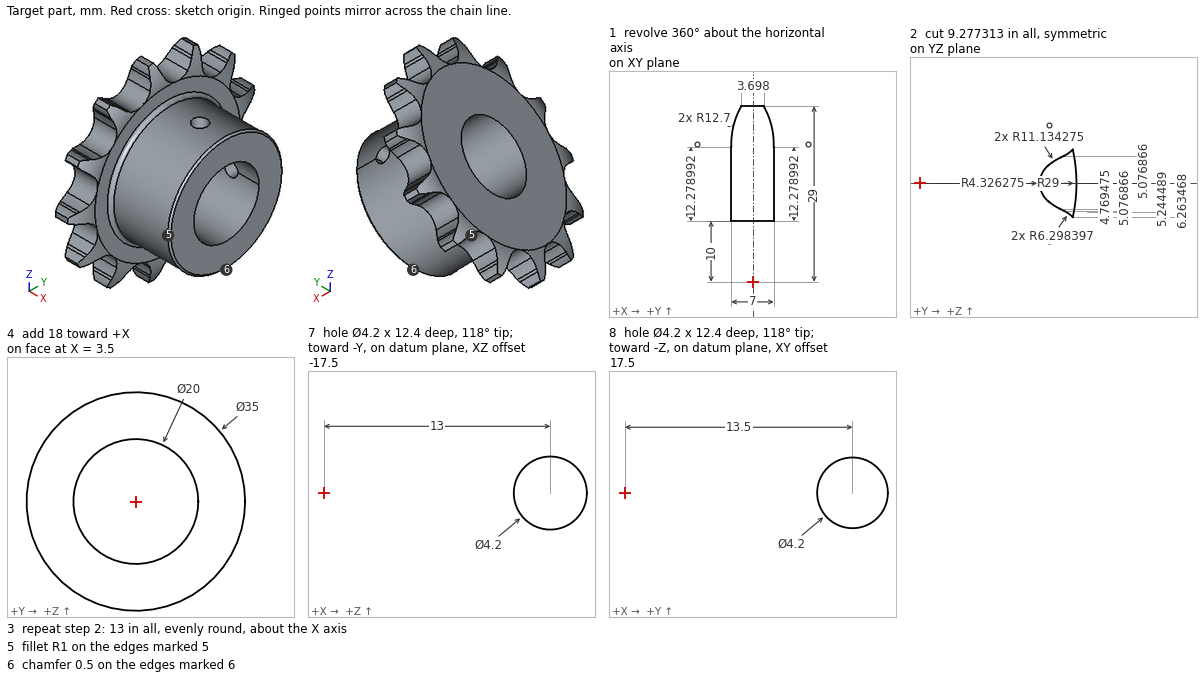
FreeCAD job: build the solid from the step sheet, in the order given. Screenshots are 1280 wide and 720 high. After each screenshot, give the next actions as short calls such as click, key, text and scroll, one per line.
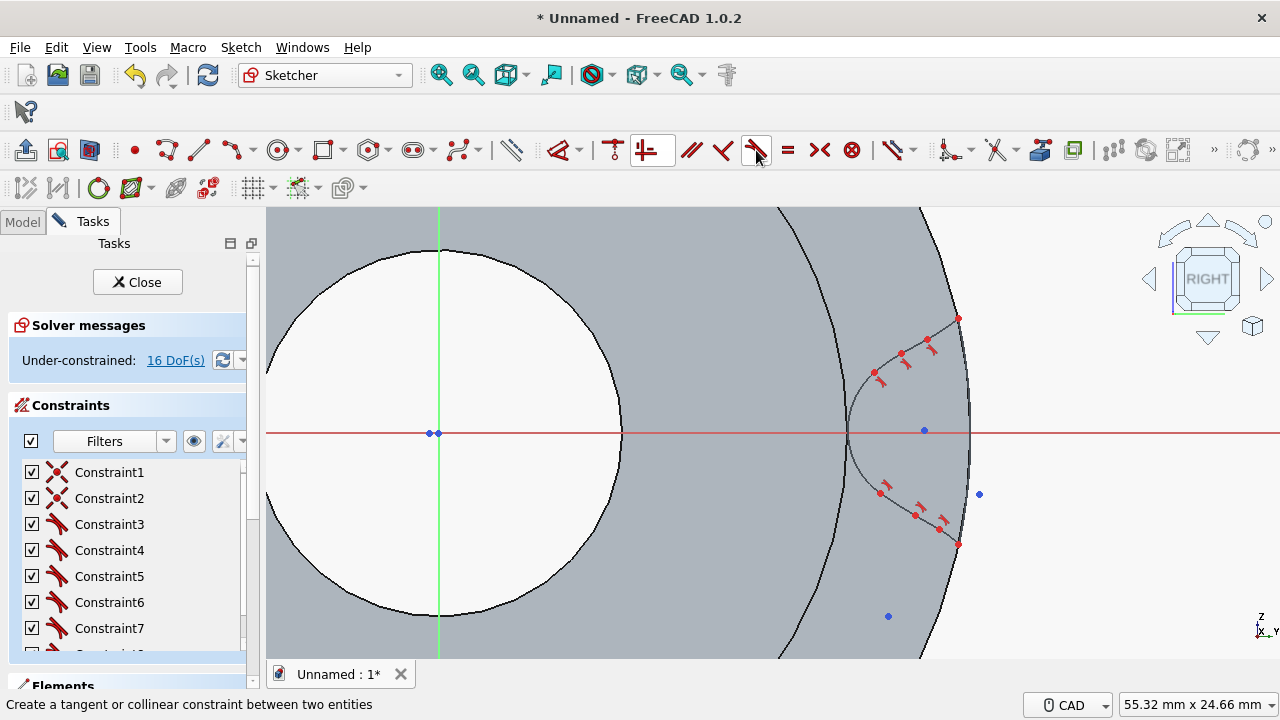
drag(419, 423, 449, 444)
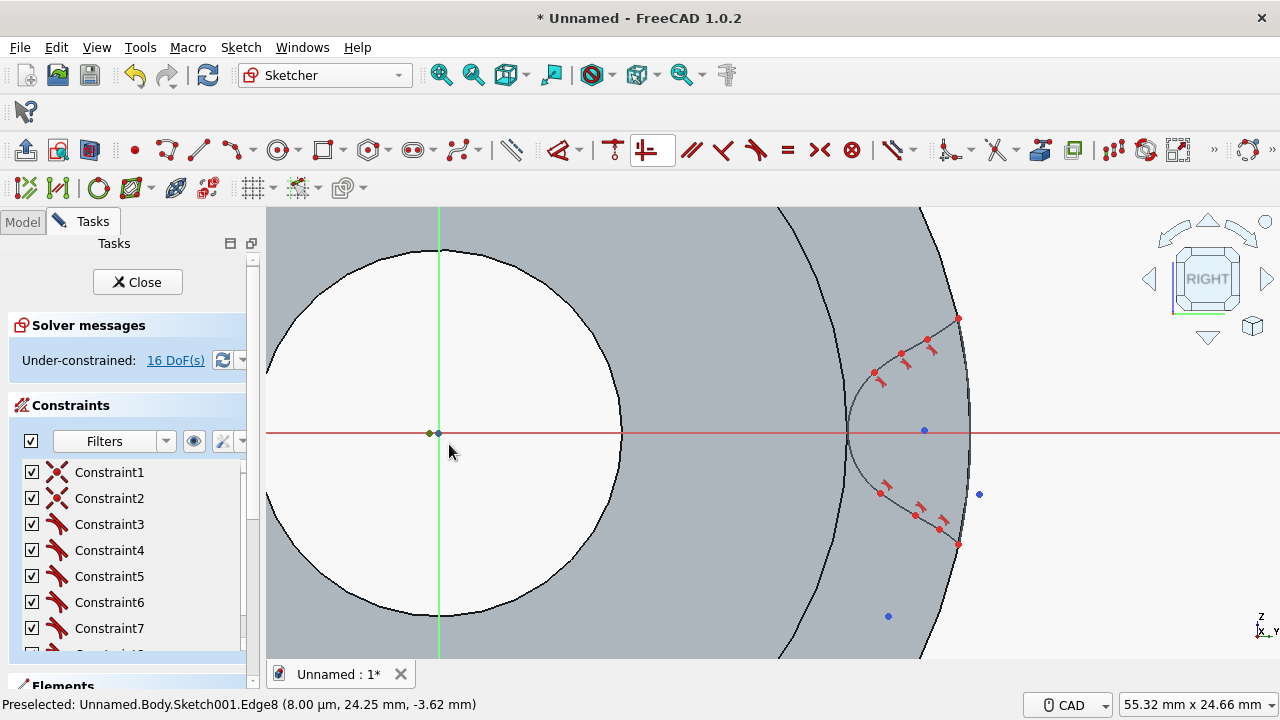
key(c)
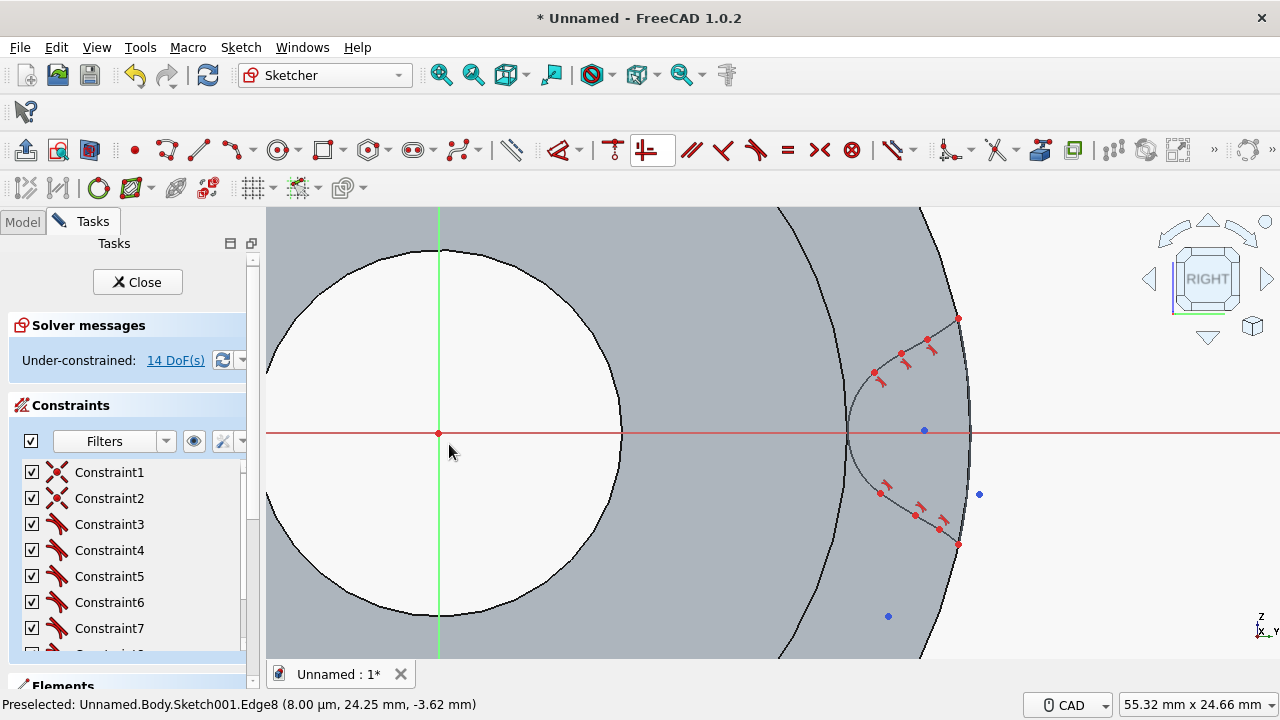
scroll(949, 536, up, 2)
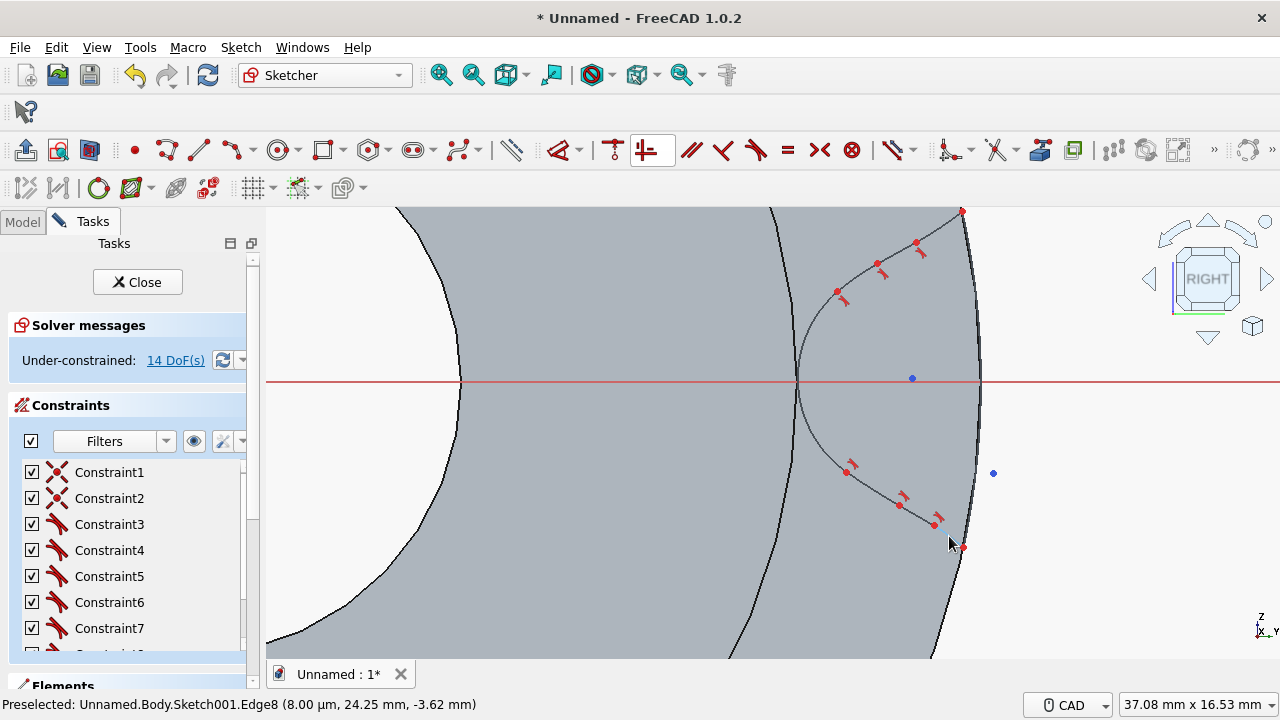
click(949, 536)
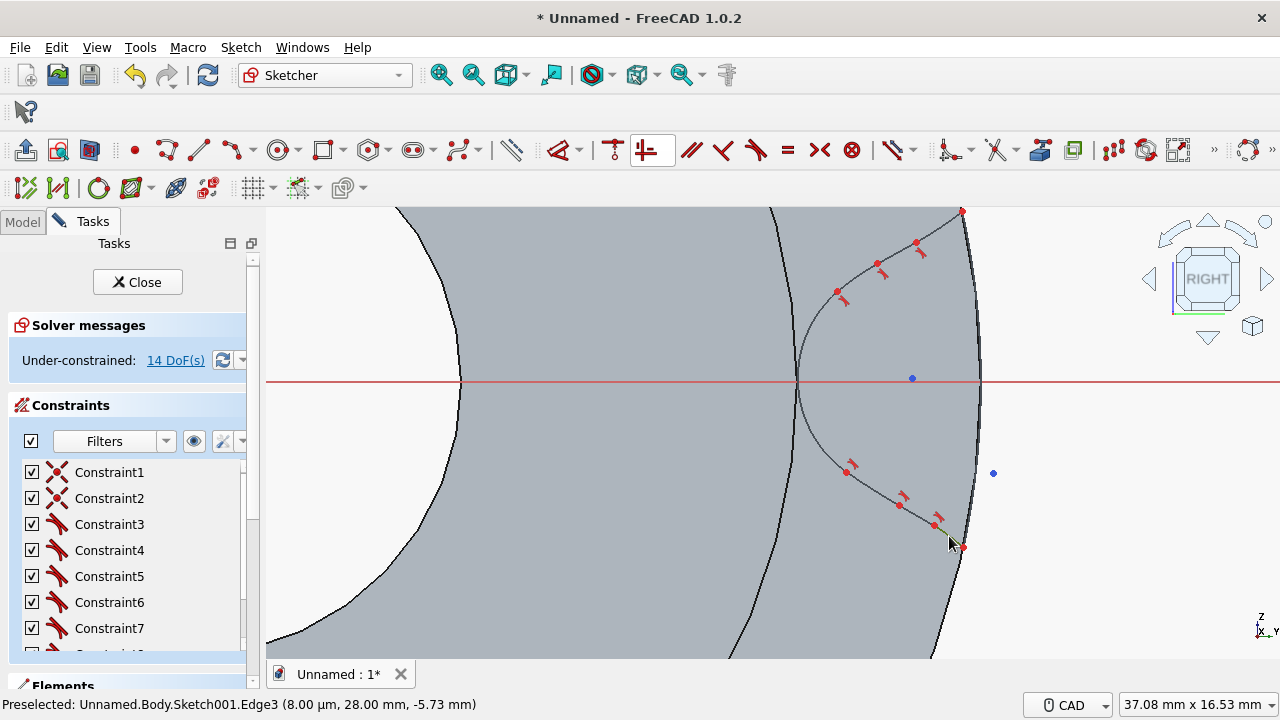
scroll(926, 237, up, 2)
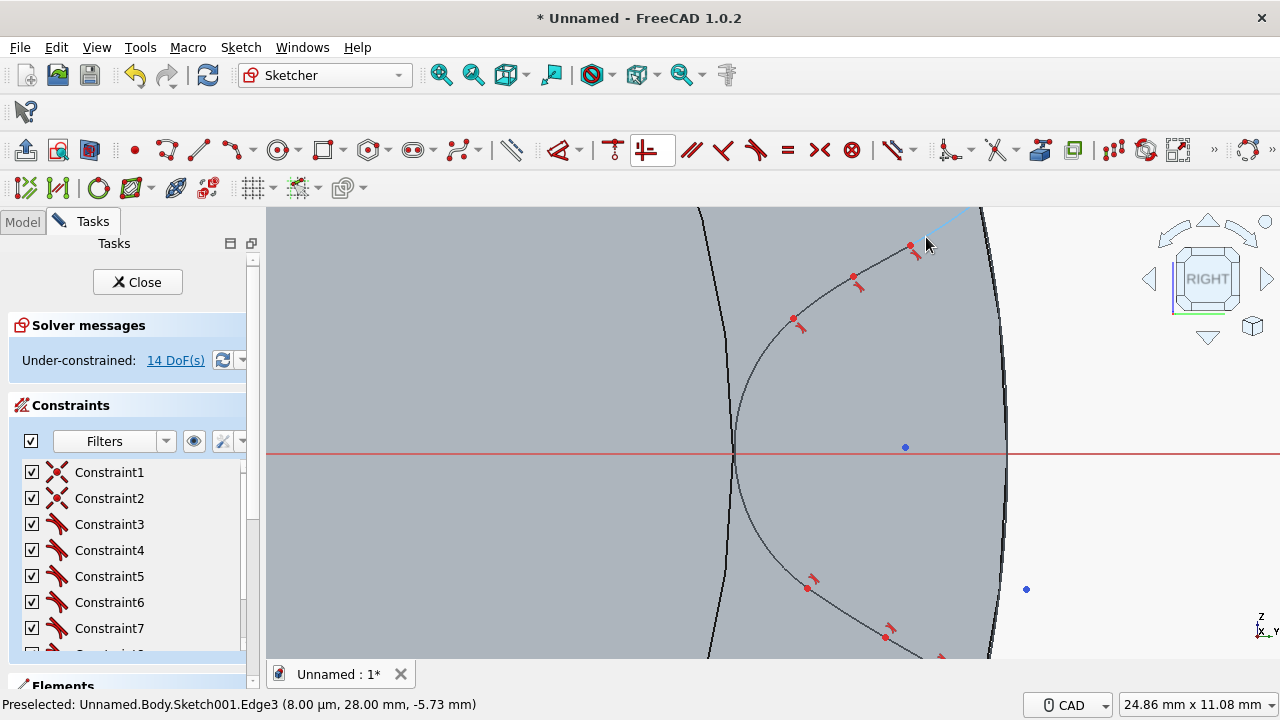
click(925, 237)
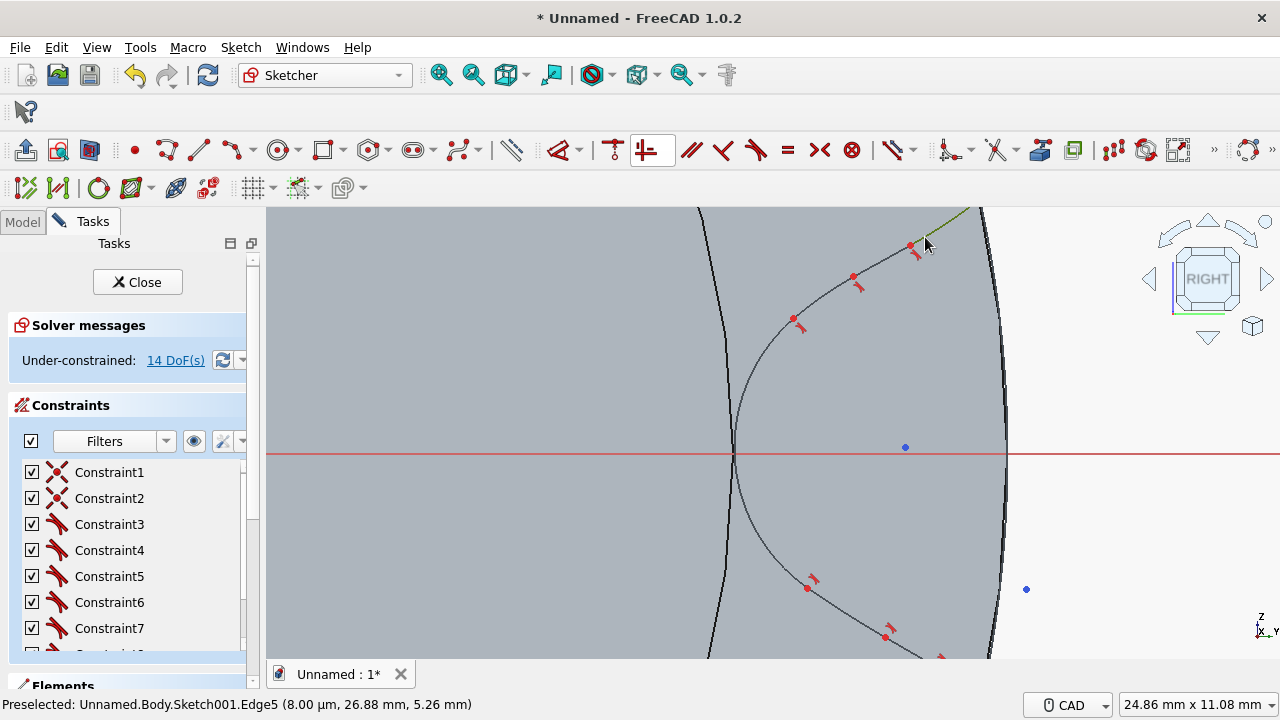
click(788, 150)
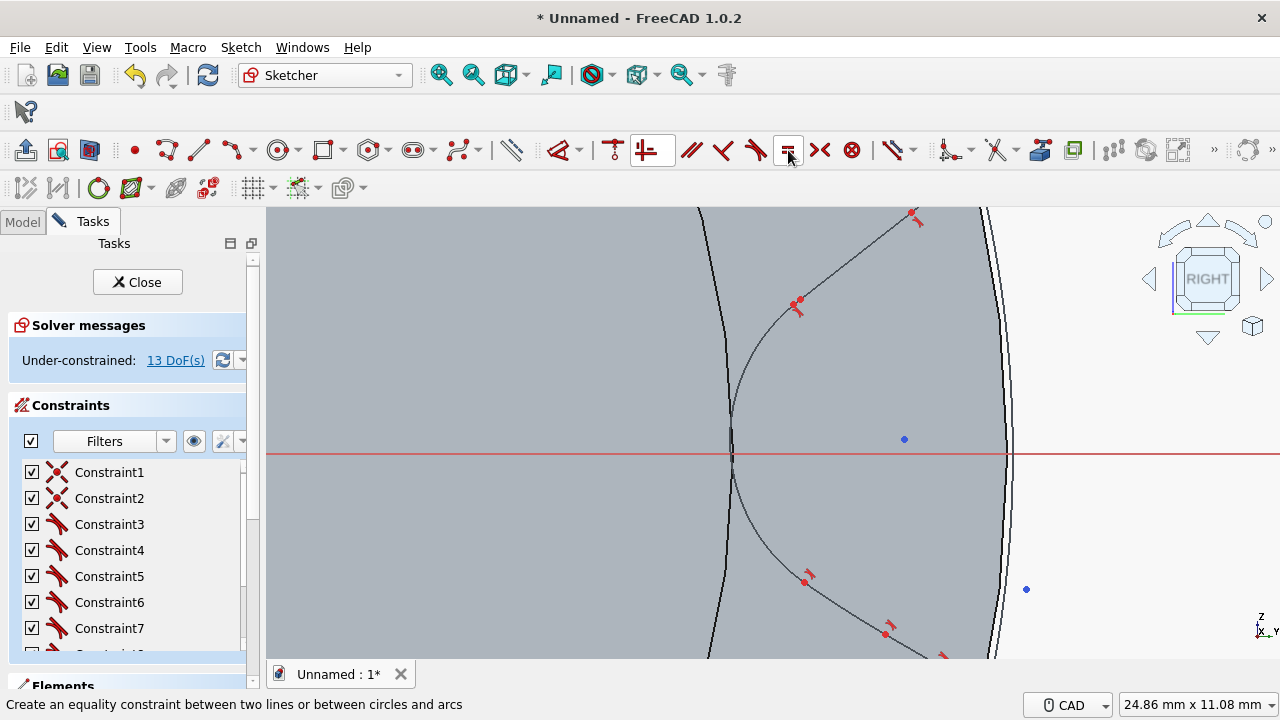
scroll(797, 302, up, 6)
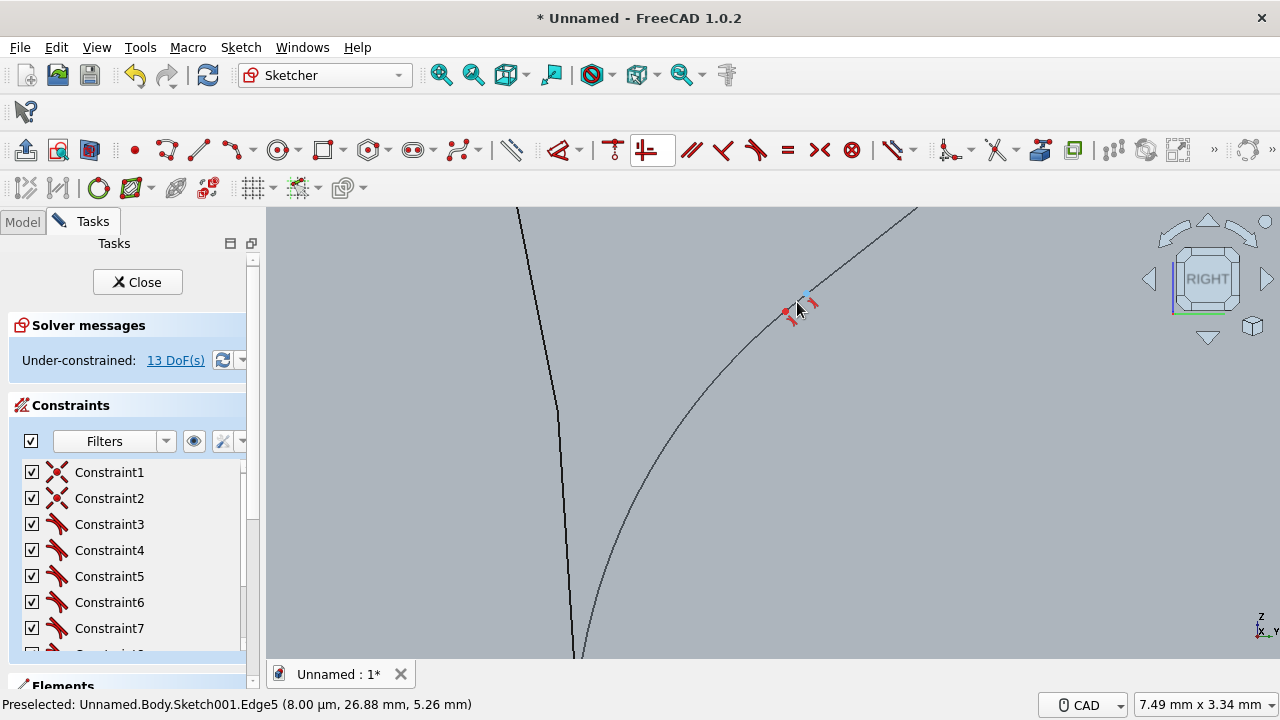
click(796, 303)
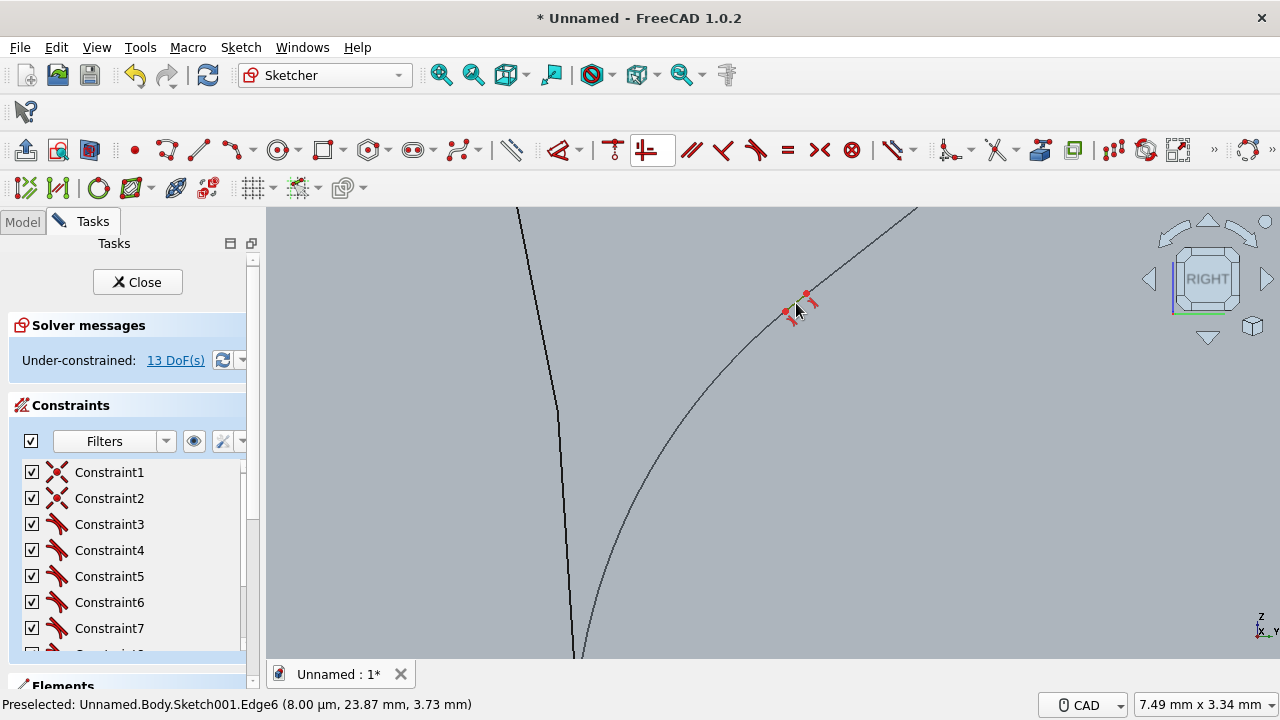
scroll(888, 375, down, 10)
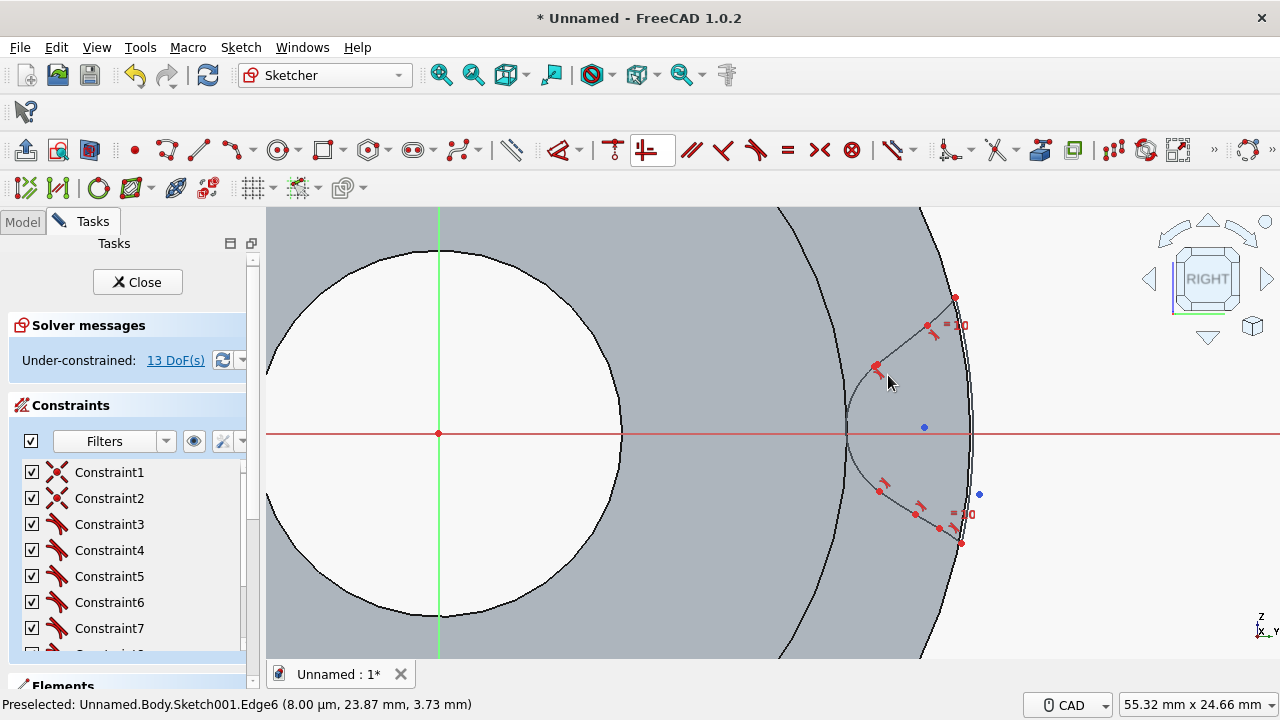
click(890, 499)